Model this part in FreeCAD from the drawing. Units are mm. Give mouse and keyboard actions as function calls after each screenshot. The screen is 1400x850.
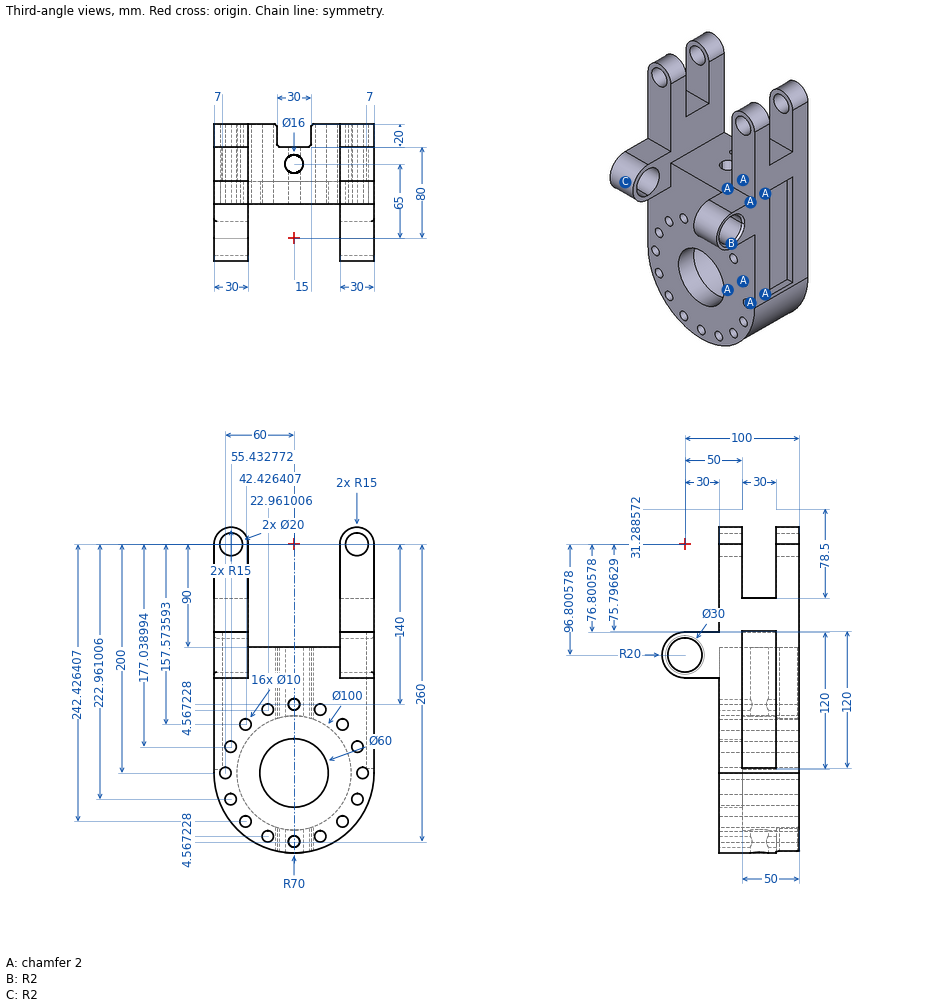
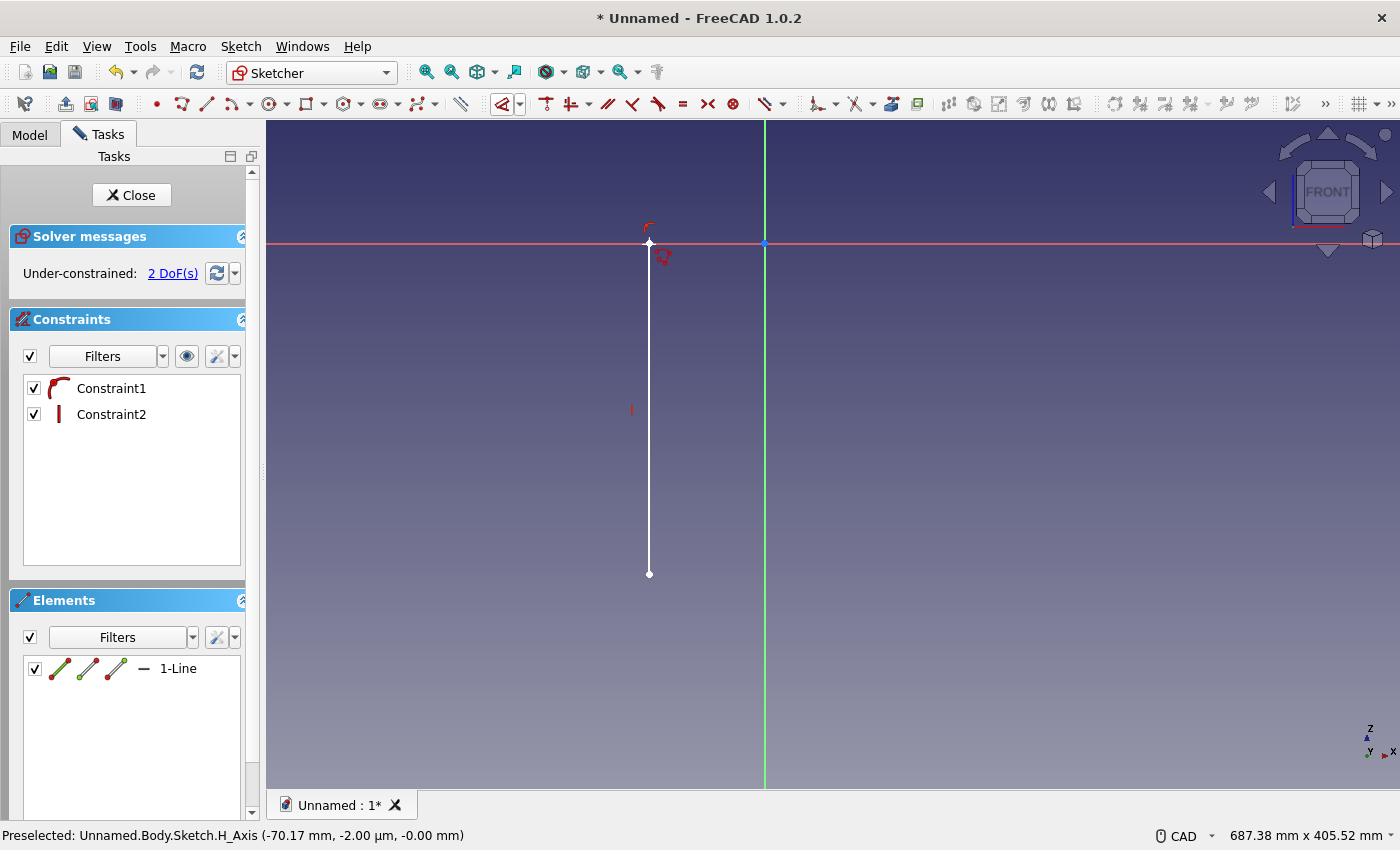
click(699, 244)
click(699, 392)
click(831, 392)
click(831, 244)
right_click(831, 244)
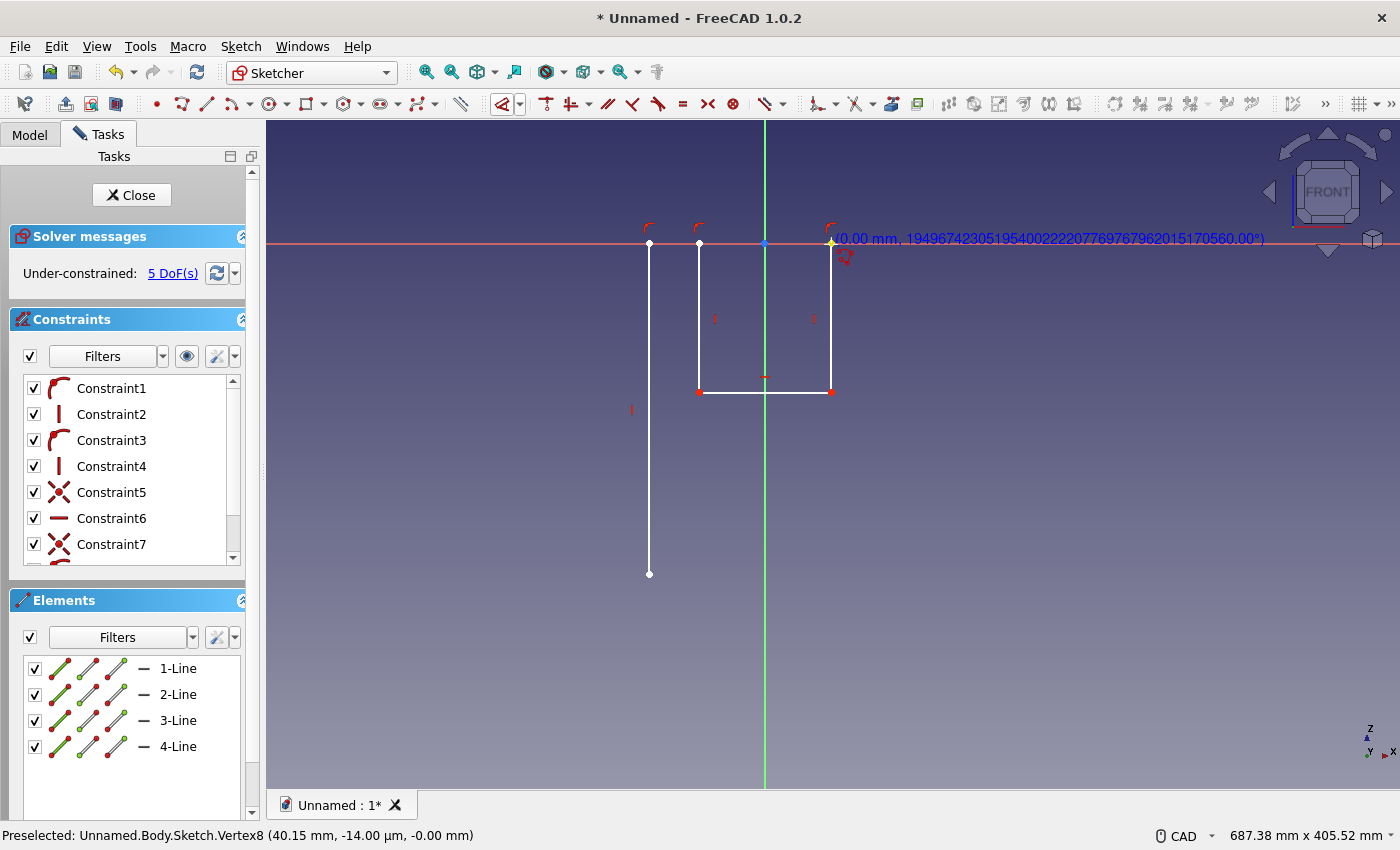
click(207, 104)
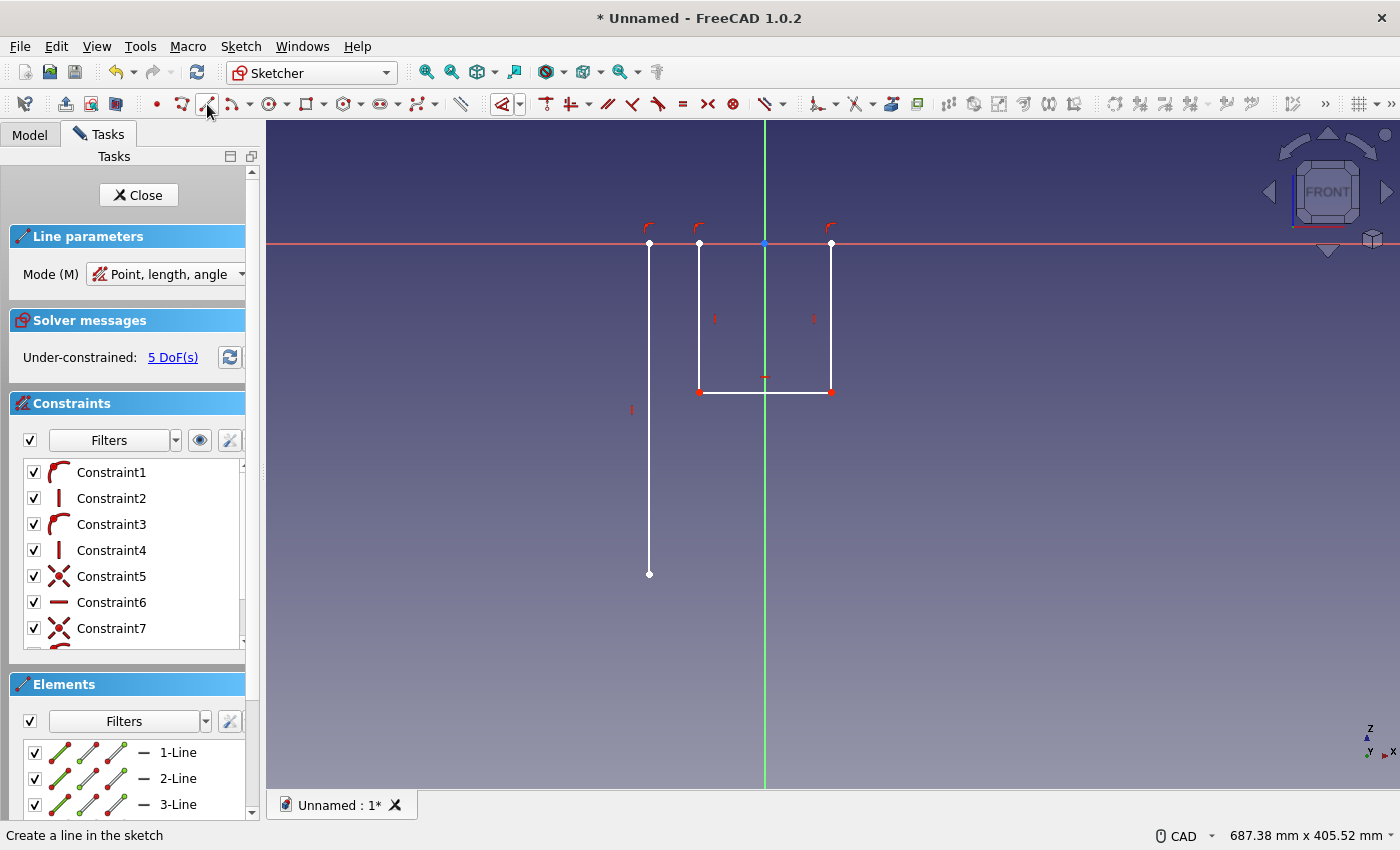
click(880, 244)
click(880, 574)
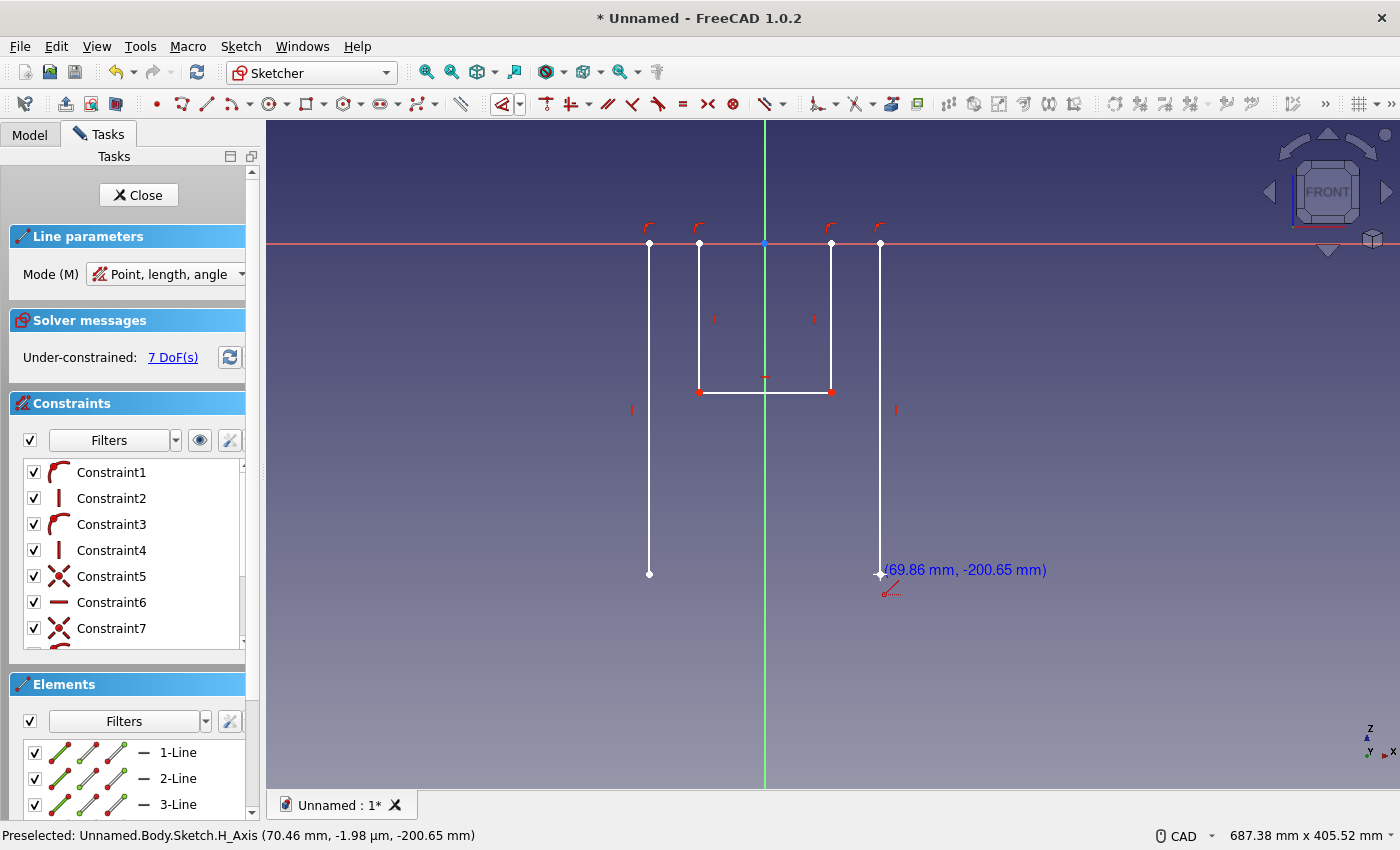
click(250, 104)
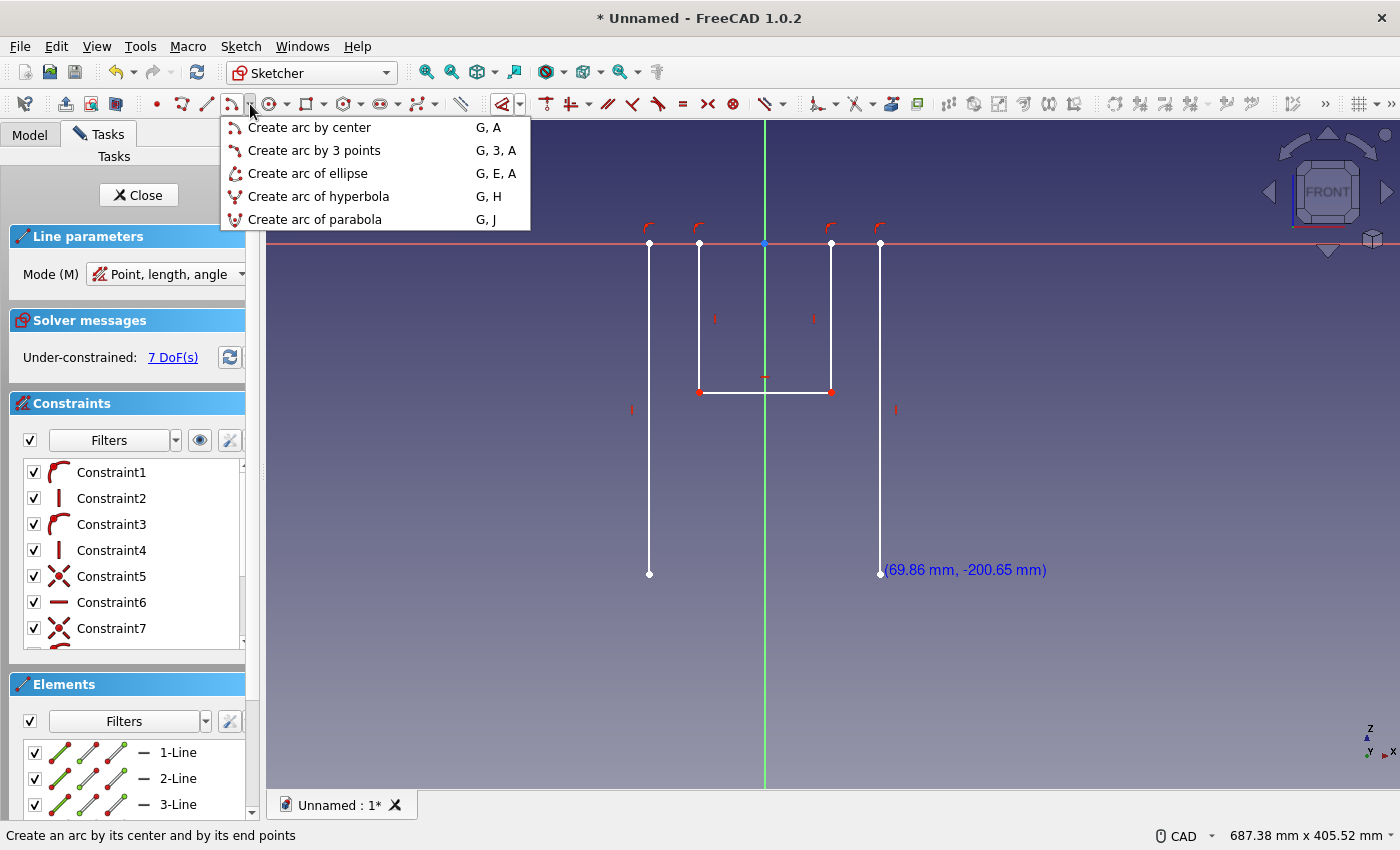
click(376, 150)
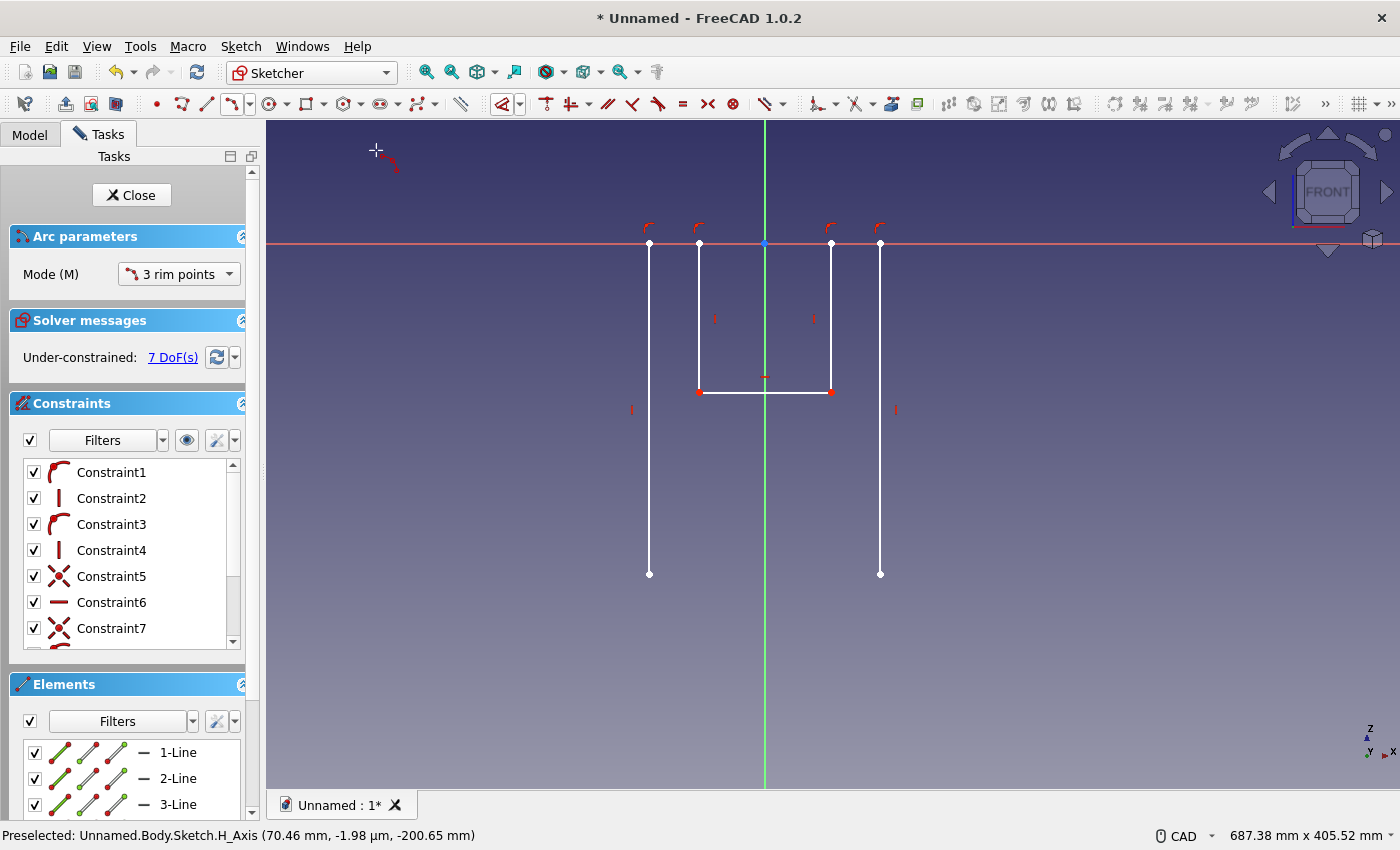
click(649, 244)
click(699, 244)
click(674, 219)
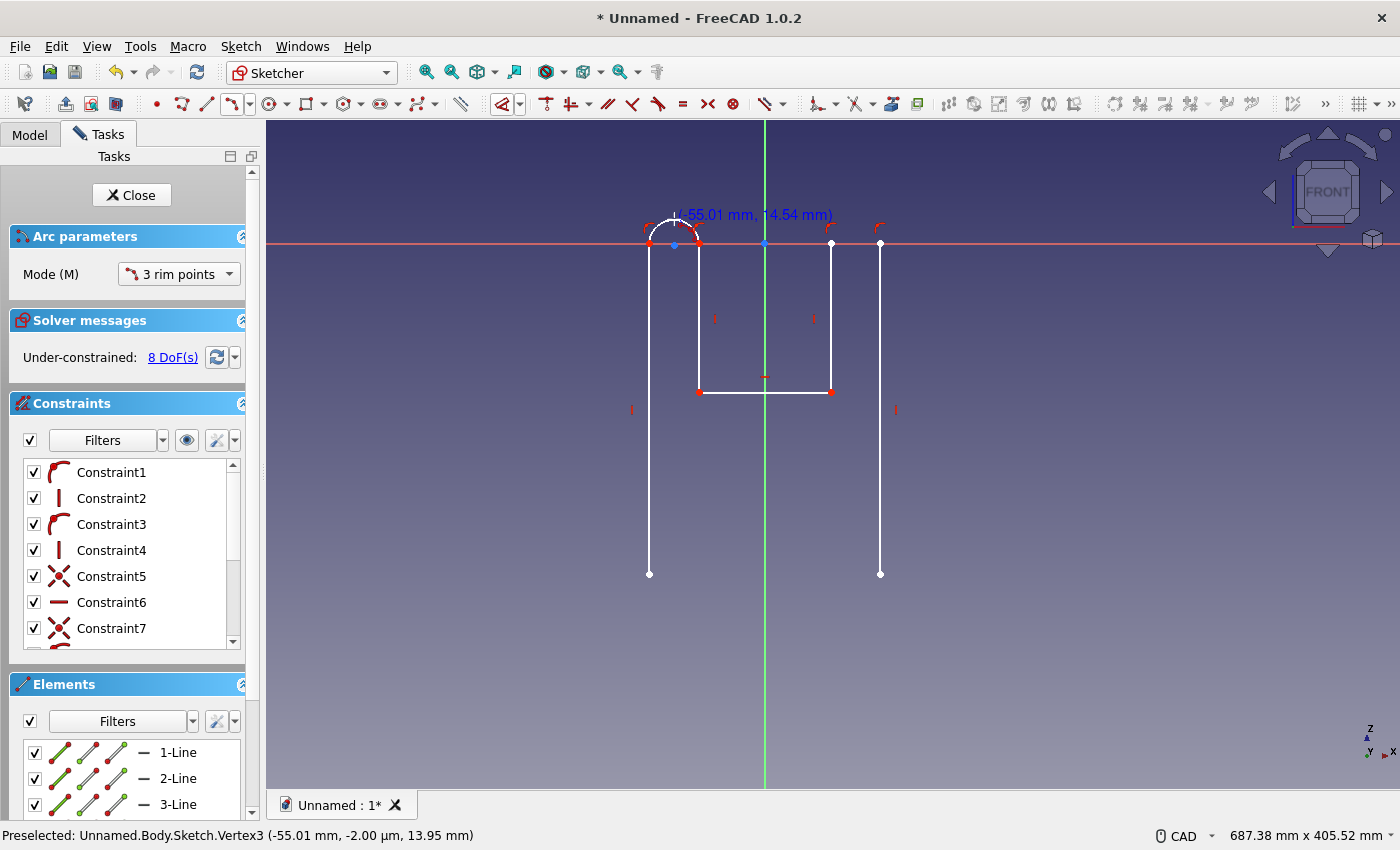
click(831, 244)
click(880, 244)
click(855, 219)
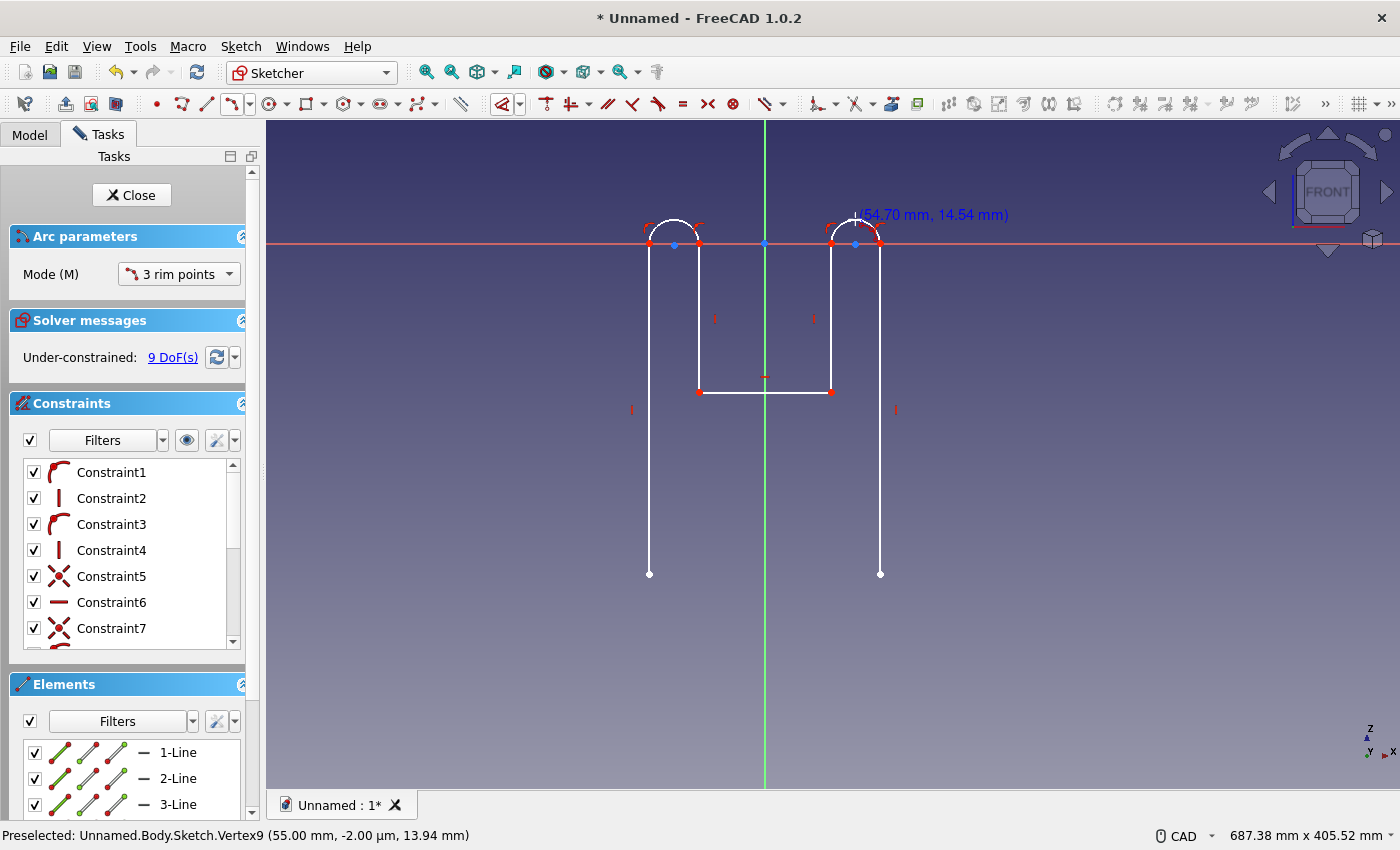
click(880, 575)
click(649, 575)
click(729, 684)